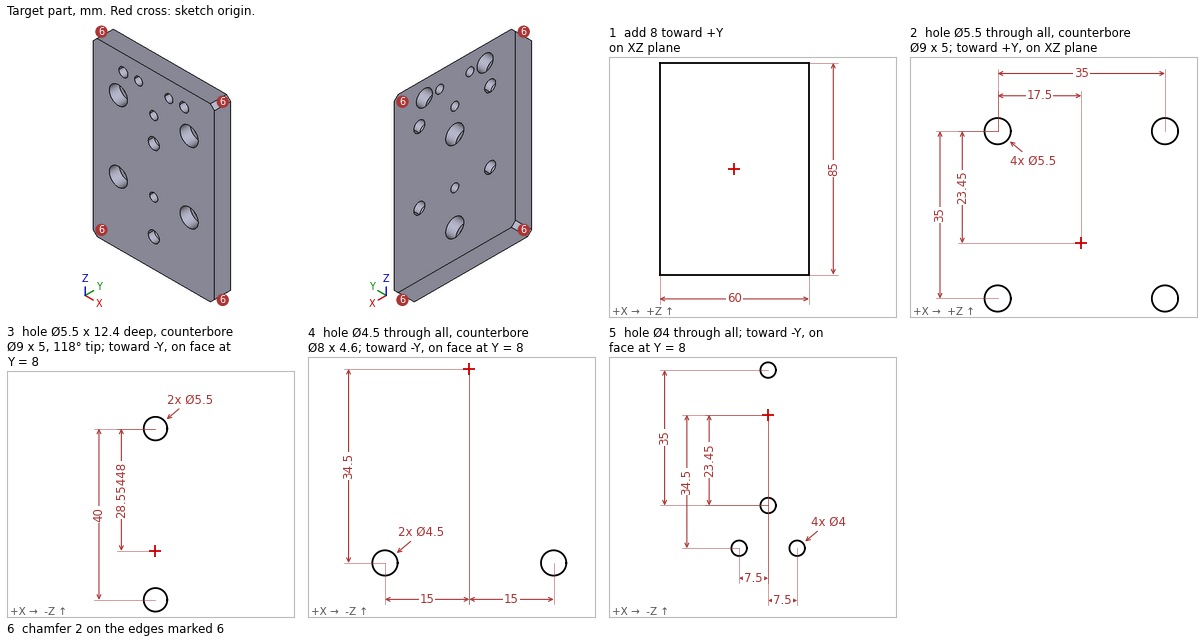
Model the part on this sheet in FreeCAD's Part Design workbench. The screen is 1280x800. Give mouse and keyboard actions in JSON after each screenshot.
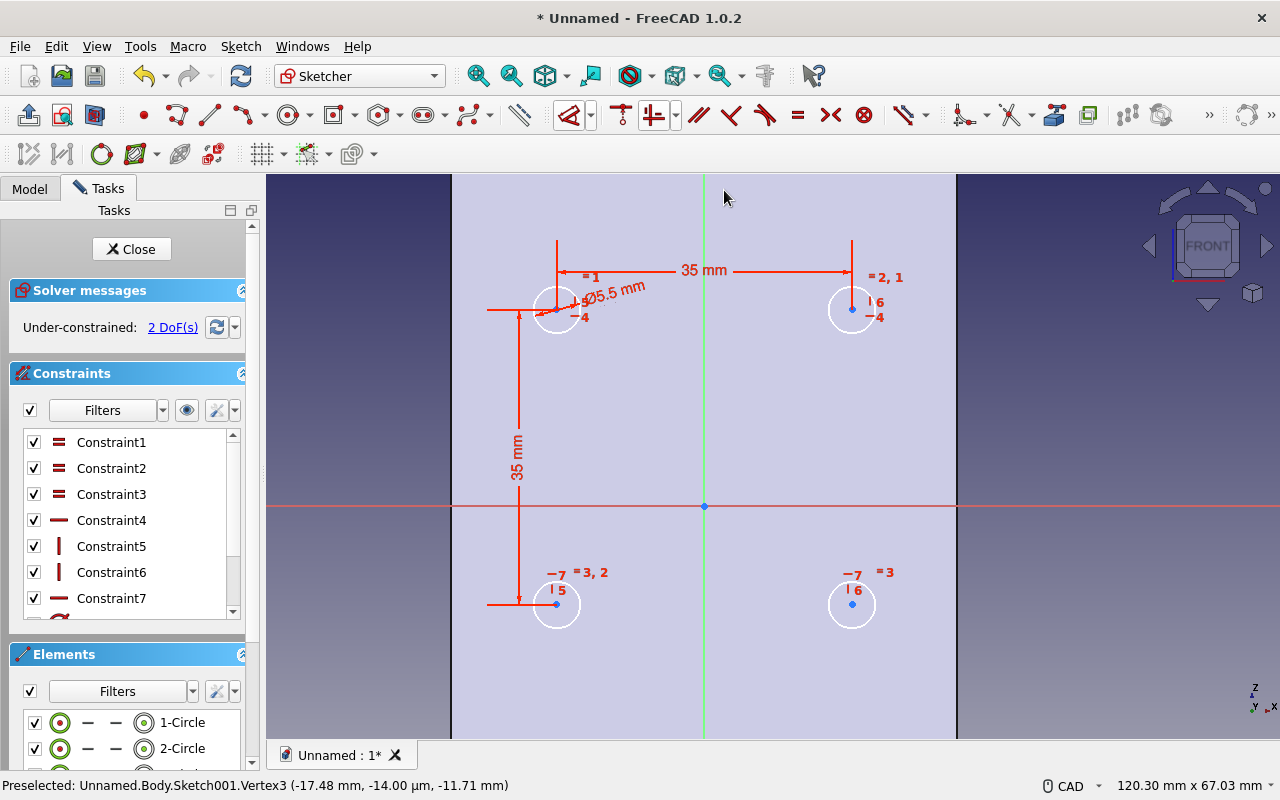
{"action": "left_click", "coordinate": [557, 310]}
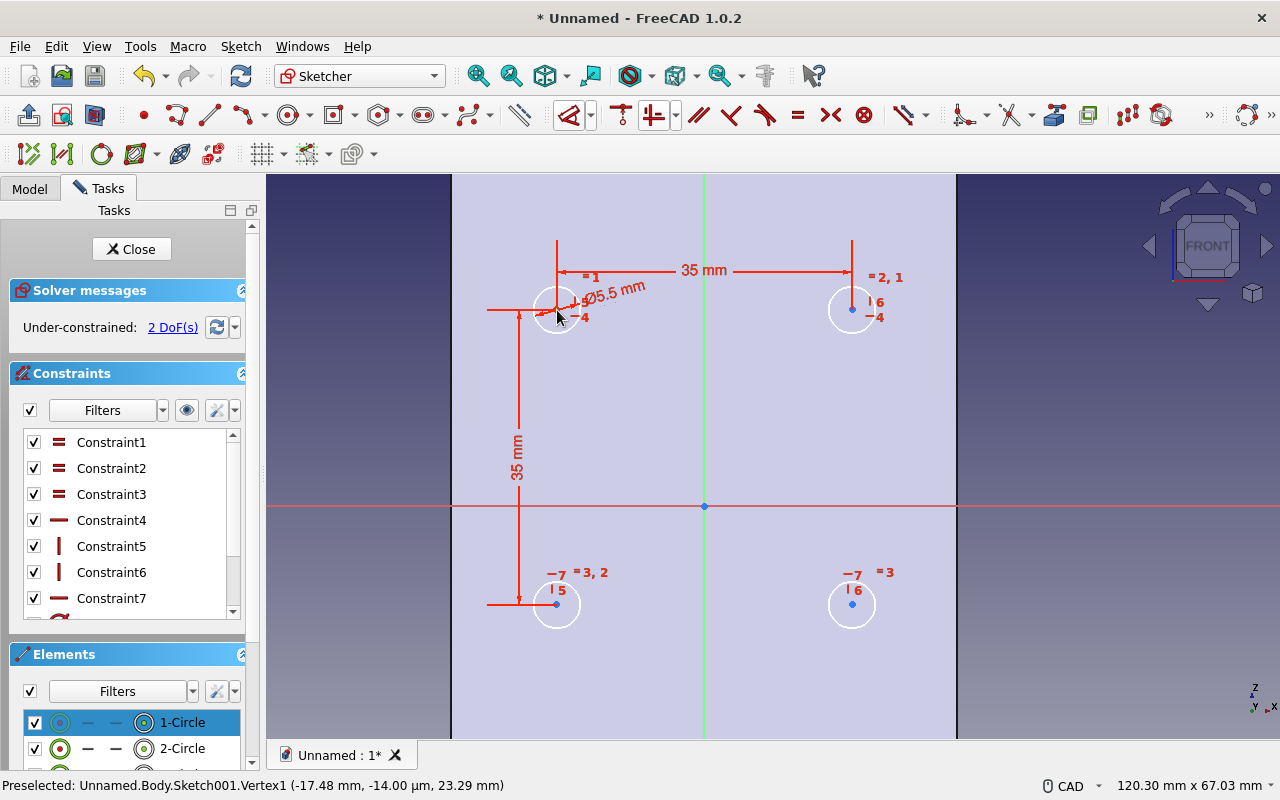
{"action": "key", "text": "l"}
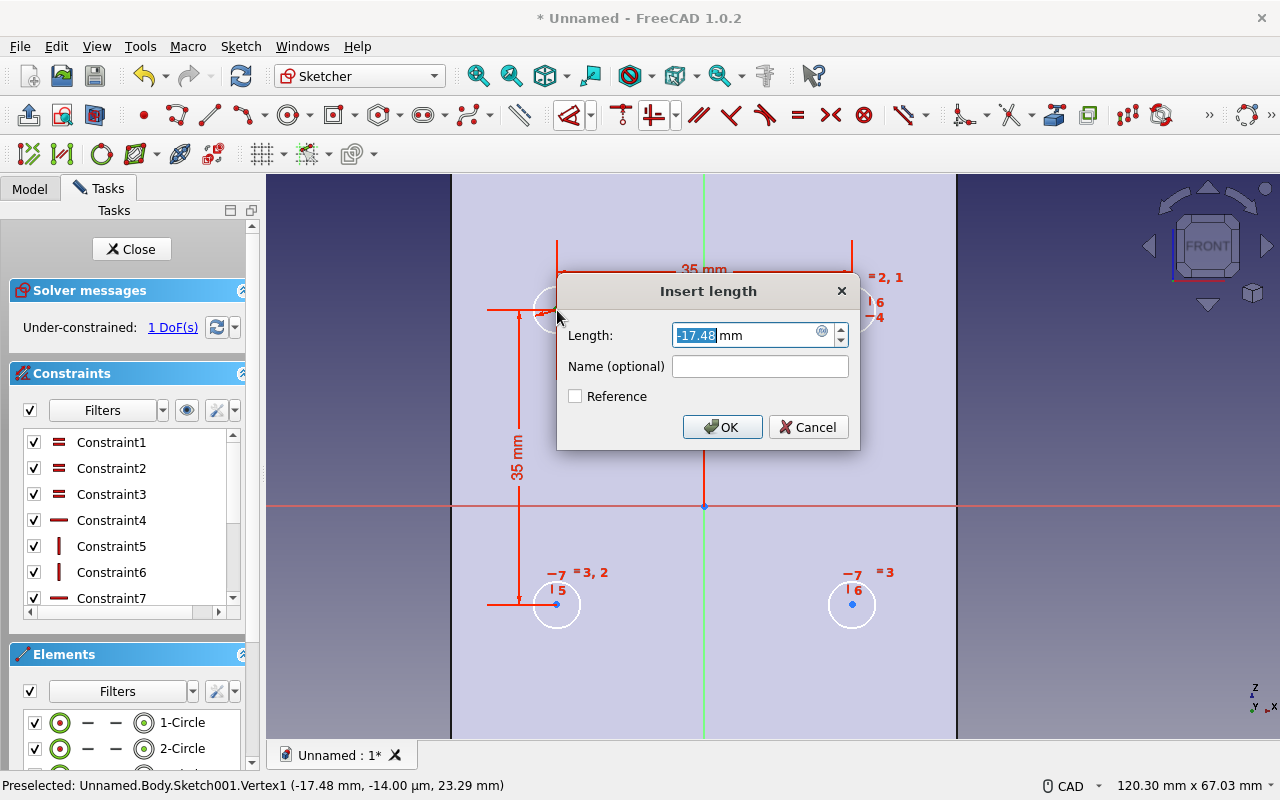
{"action": "type", "text": "-17.5"}
{"action": "key", "text": "Return"}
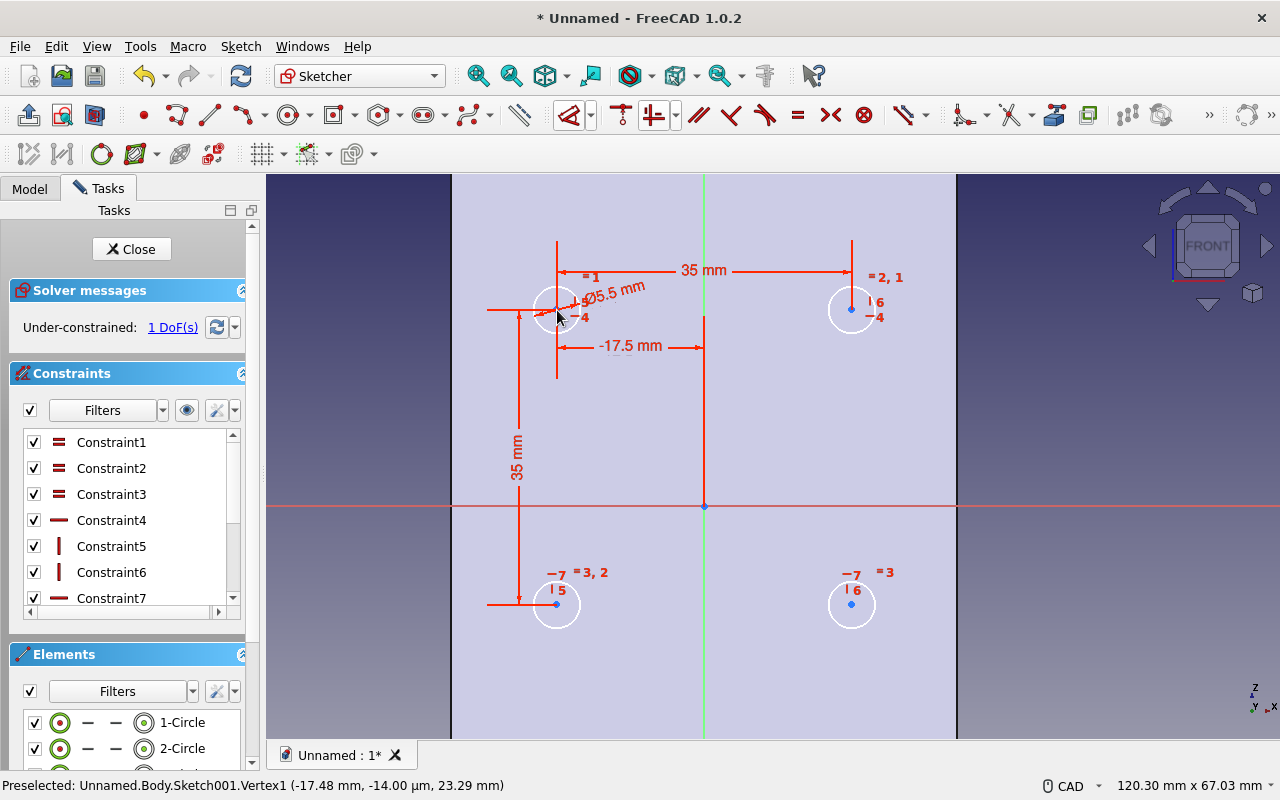
{"action": "left_click", "coordinate": [557, 310]}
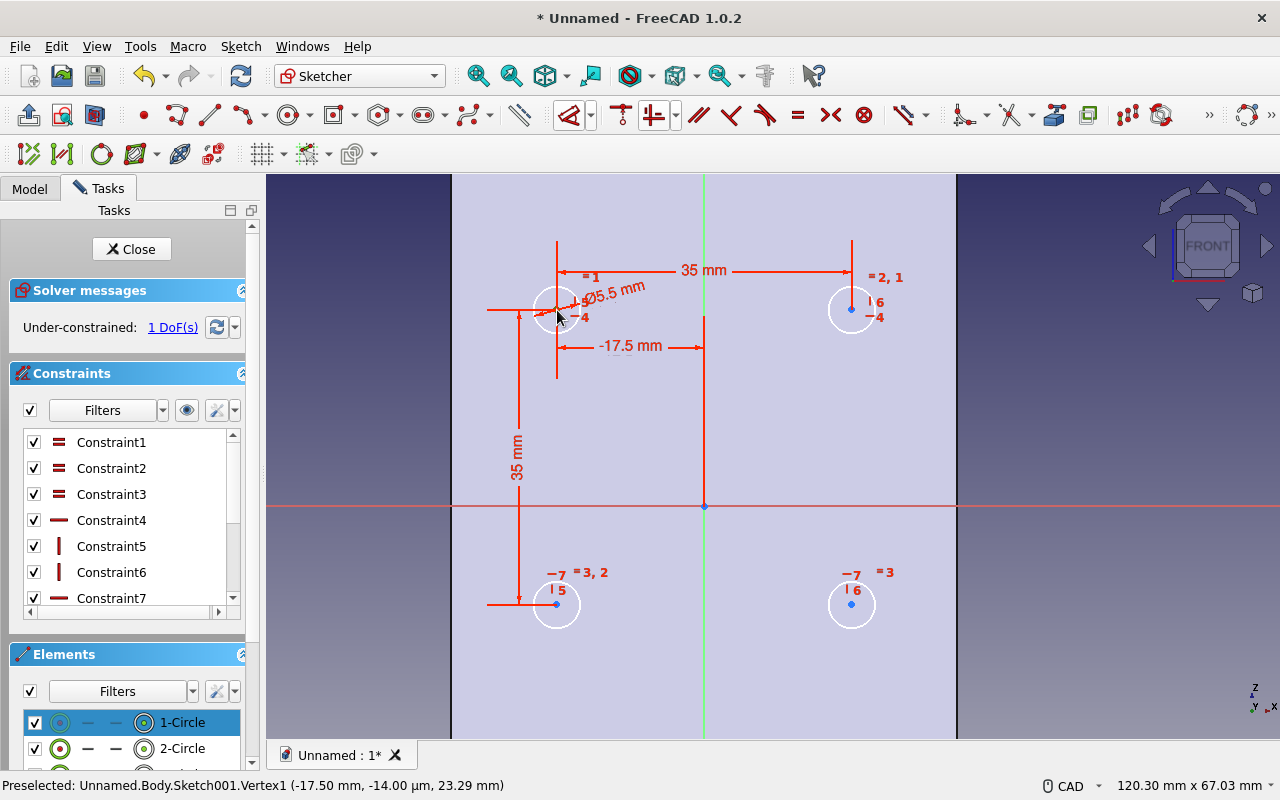
{"action": "key", "text": "i"}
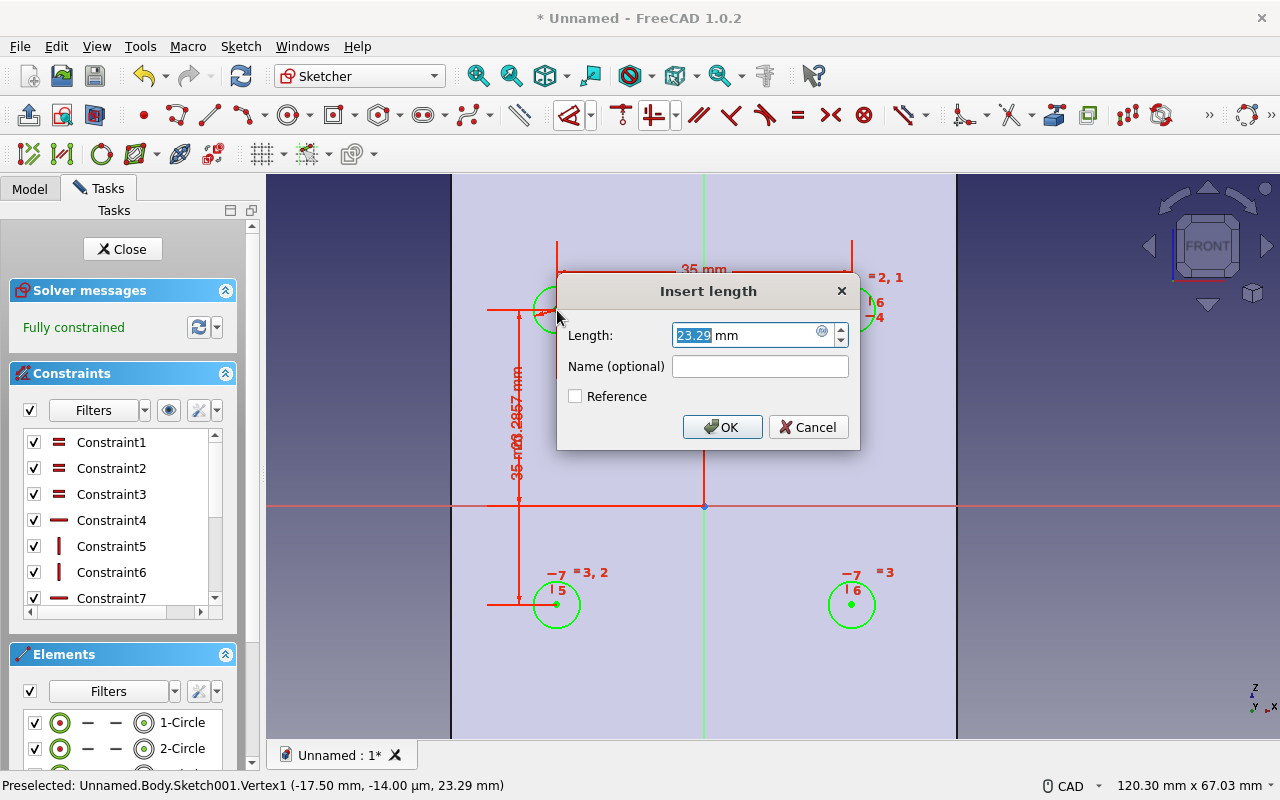
{"action": "type", "text": "23.45"}
{"action": "key", "text": "Return"}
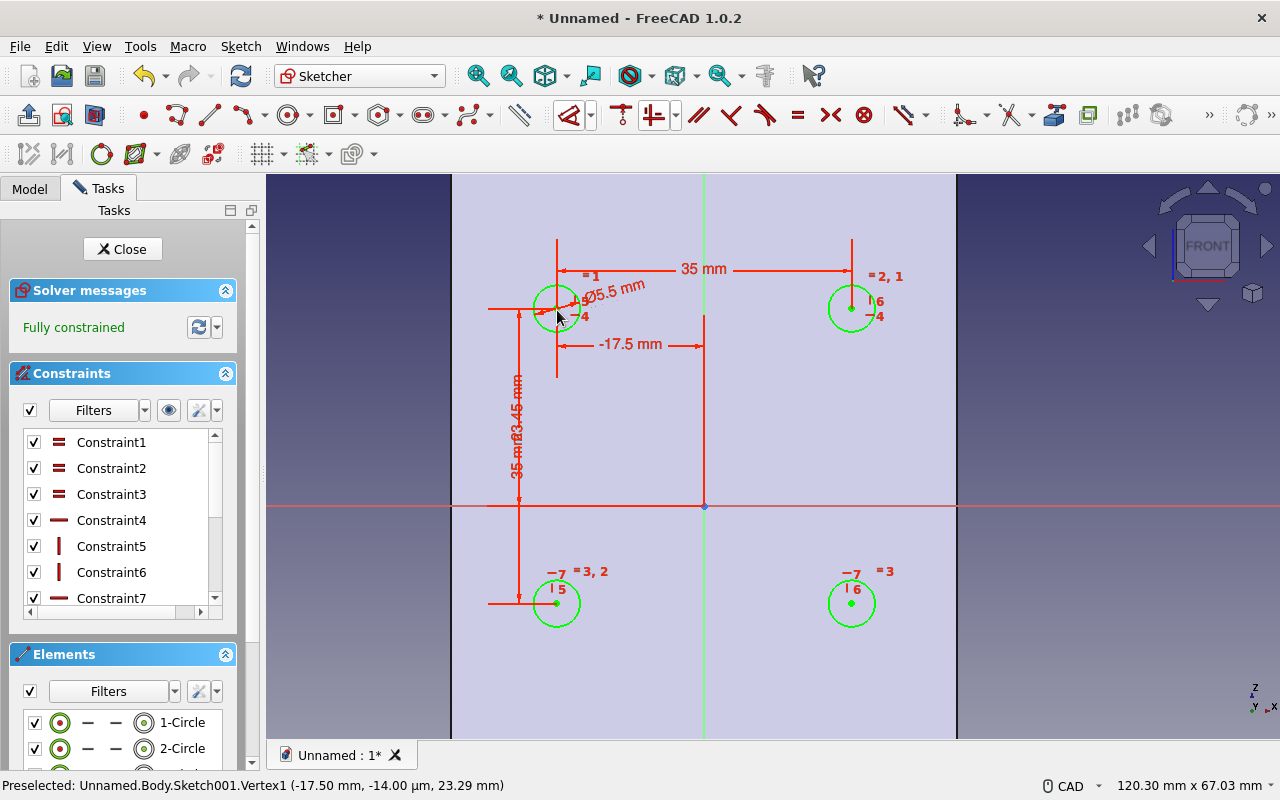
{"action": "left_click", "coordinate": [123, 249]}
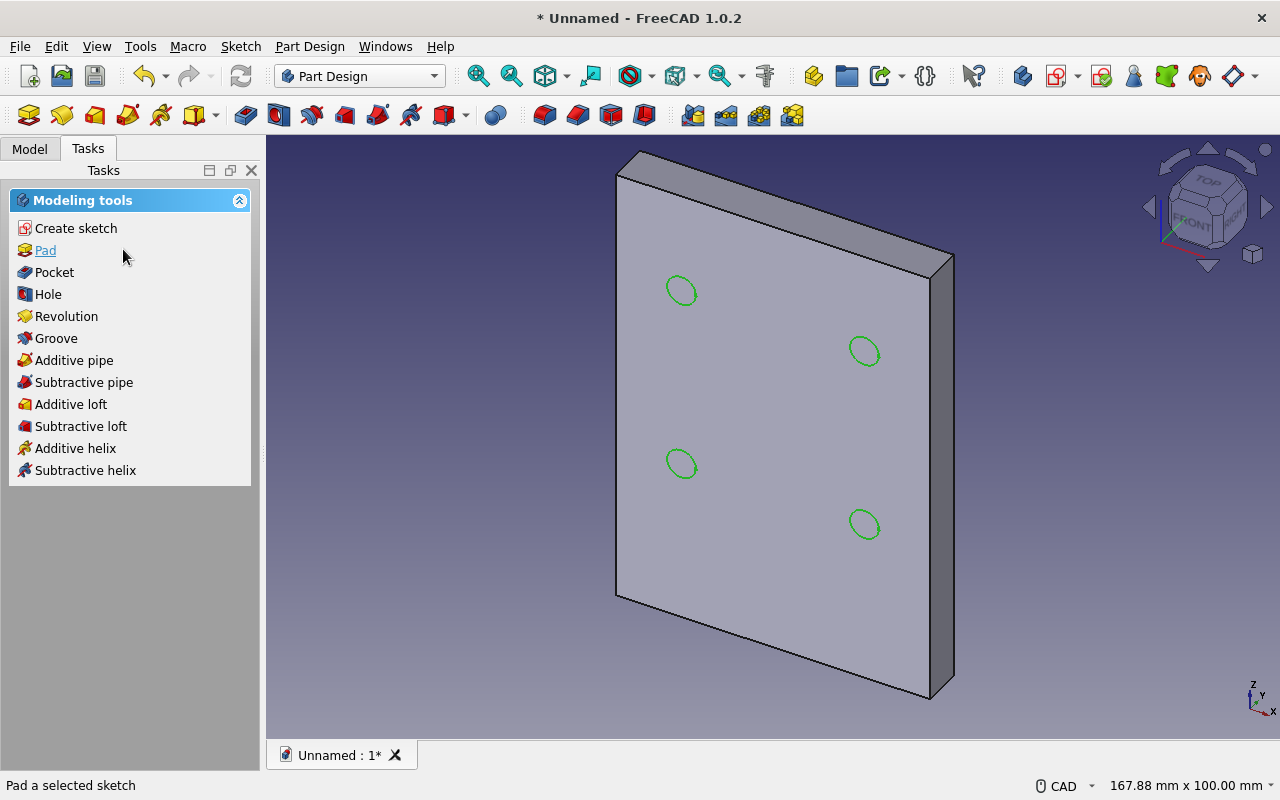
{"action": "left_click", "coordinate": [279, 116]}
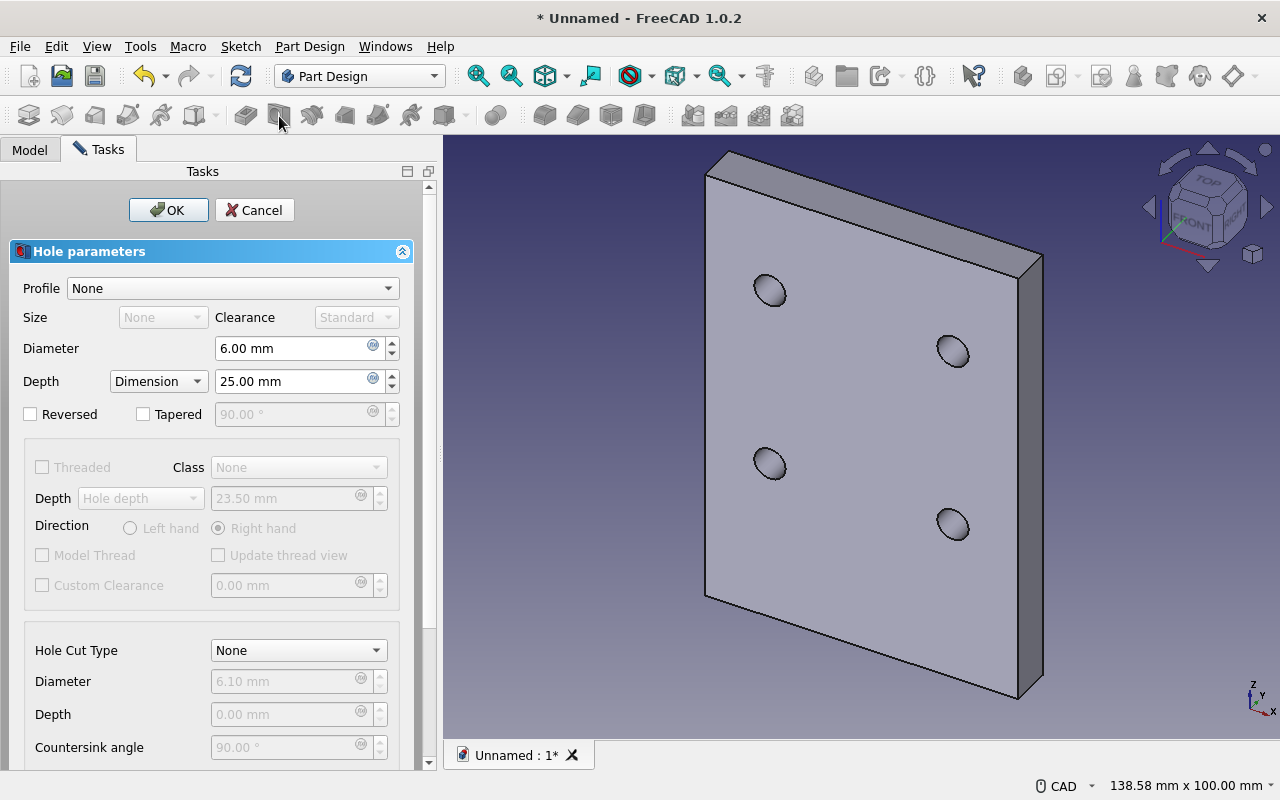
{"action": "triple_click", "coordinate": [300, 348]}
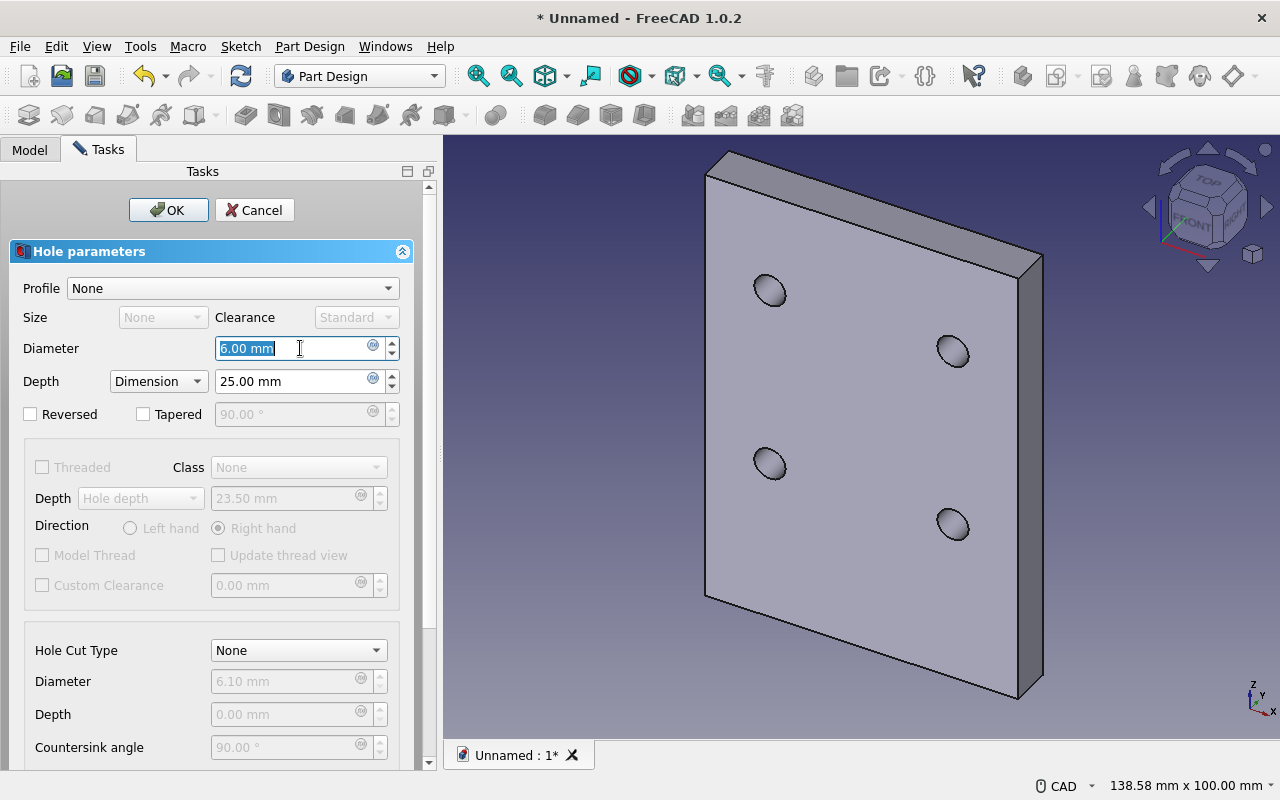
{"action": "type", "text": "5.5"}
{"action": "key", "text": "Tab"}